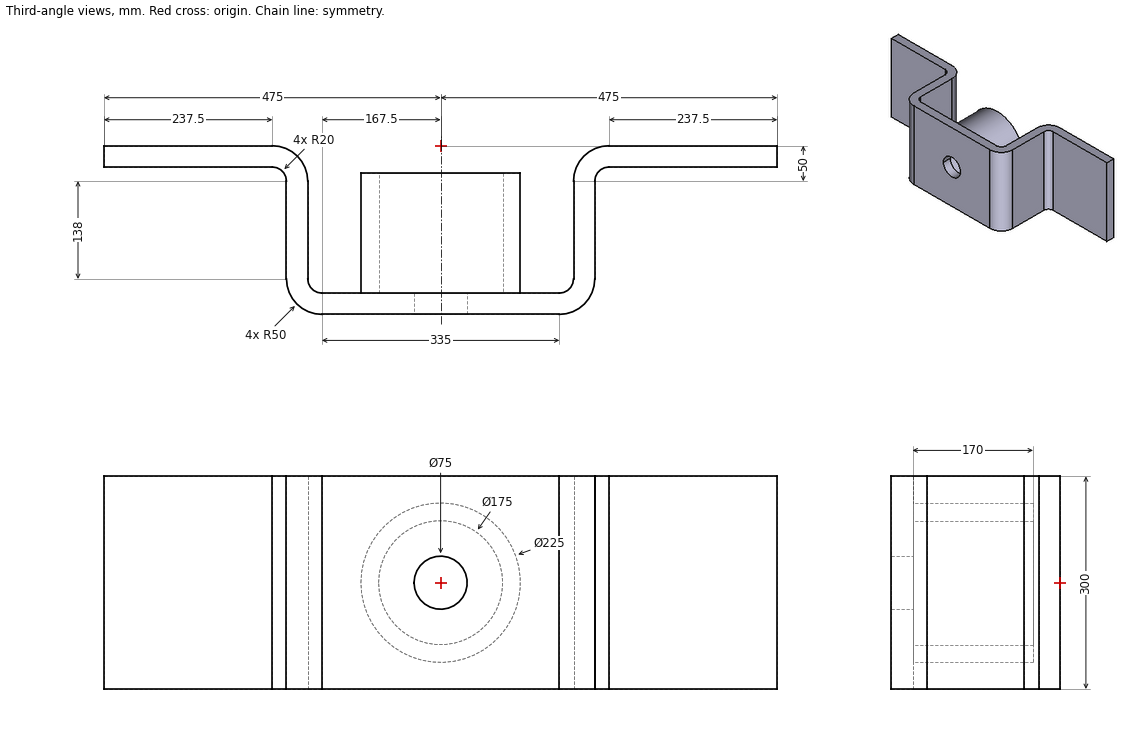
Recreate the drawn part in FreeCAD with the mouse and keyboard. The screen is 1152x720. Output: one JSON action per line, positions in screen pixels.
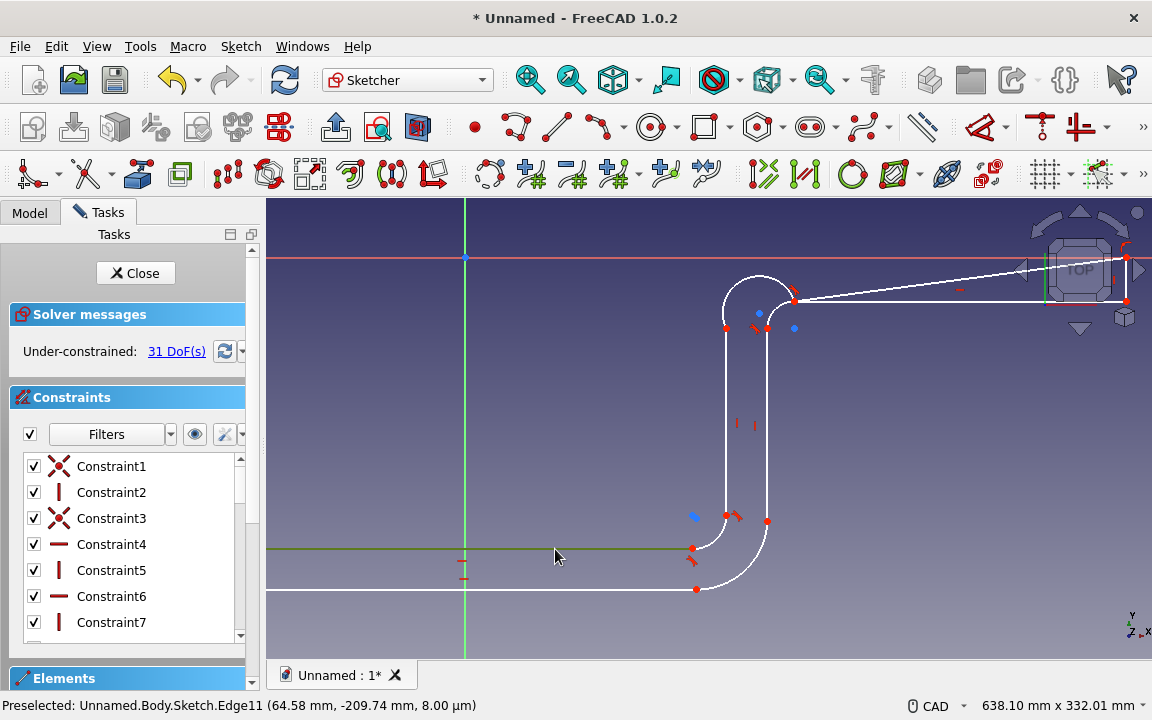
{"action": "scroll", "coordinate": [742, 432], "scroll_direction": "down", "scroll_amount": 5}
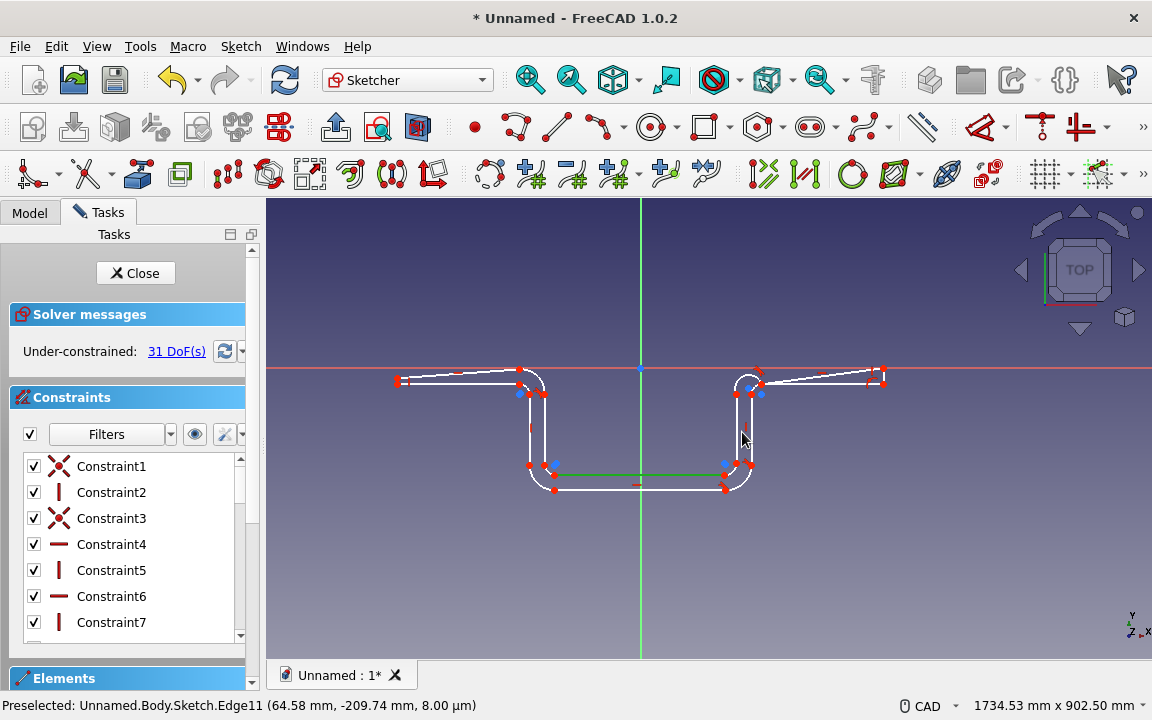
{"action": "scroll", "coordinate": [546, 470], "scroll_direction": "up", "scroll_amount": 6}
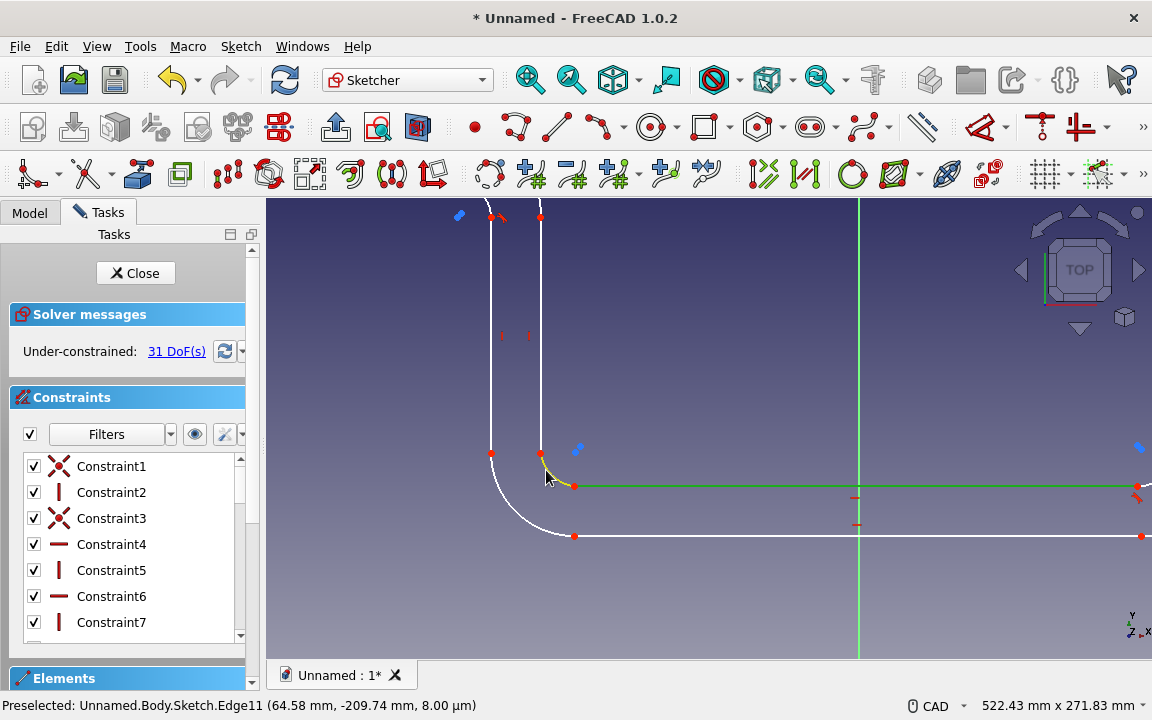
{"action": "left_click", "coordinate": [546, 467]}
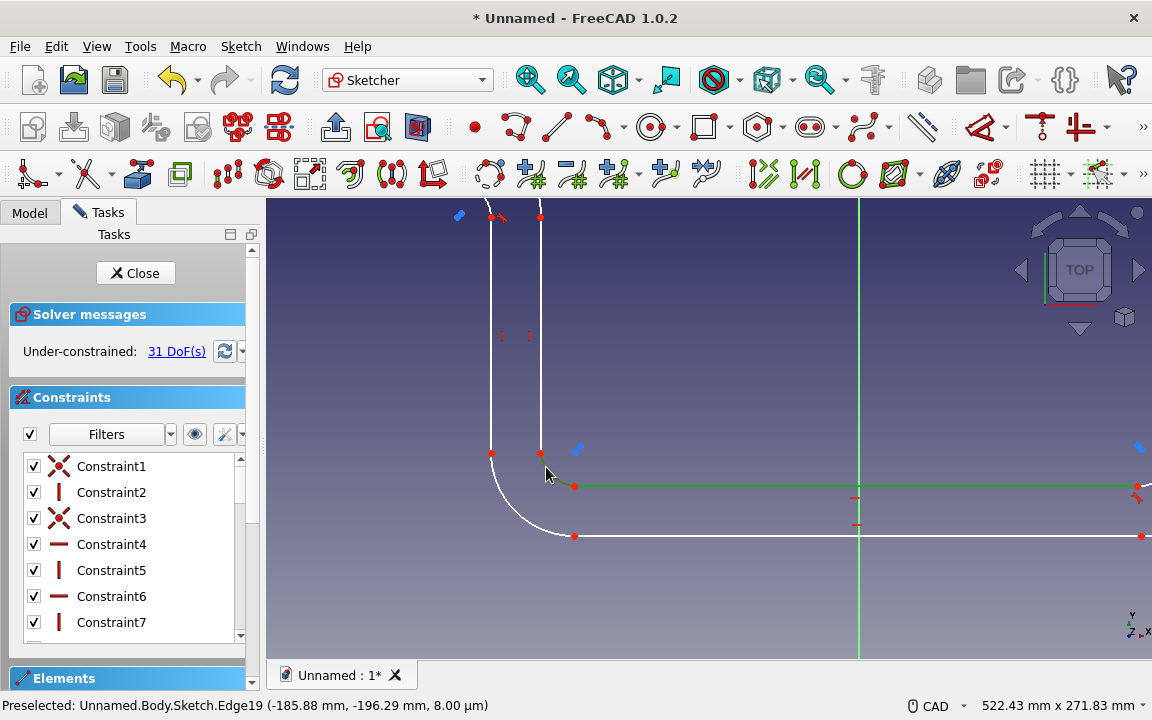
{"action": "key", "text": "t"}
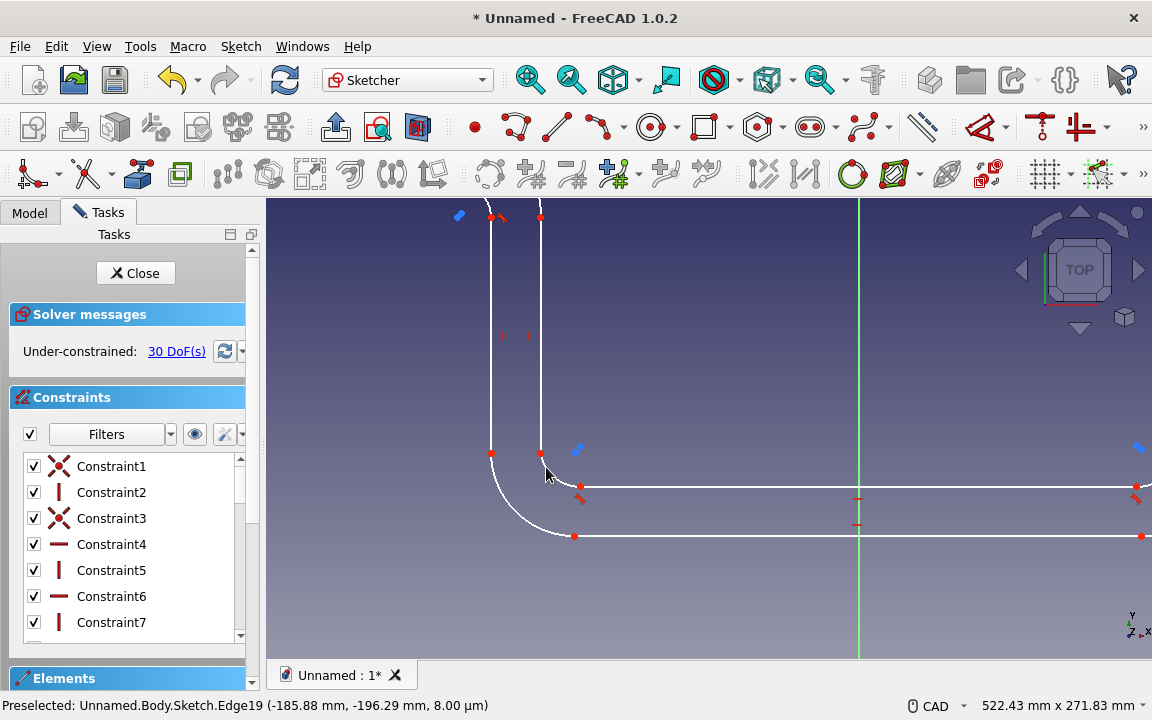
{"action": "left_click", "coordinate": [541, 382]}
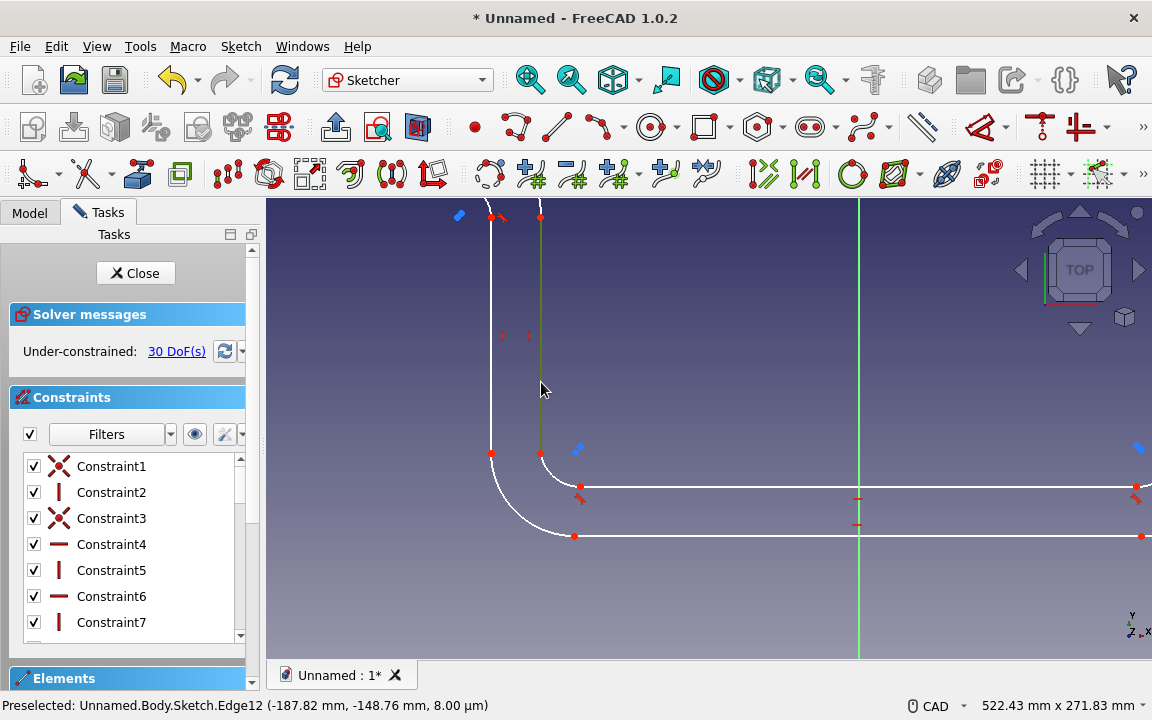
{"action": "left_click", "coordinate": [547, 469]}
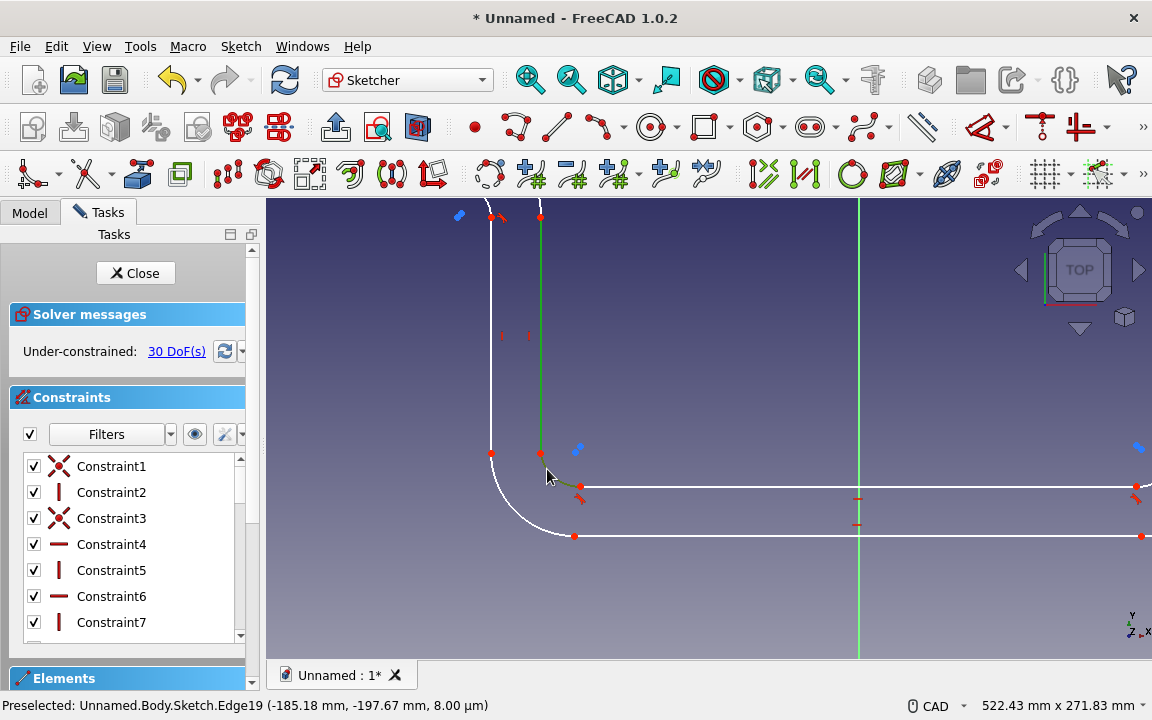
{"action": "key", "text": "t"}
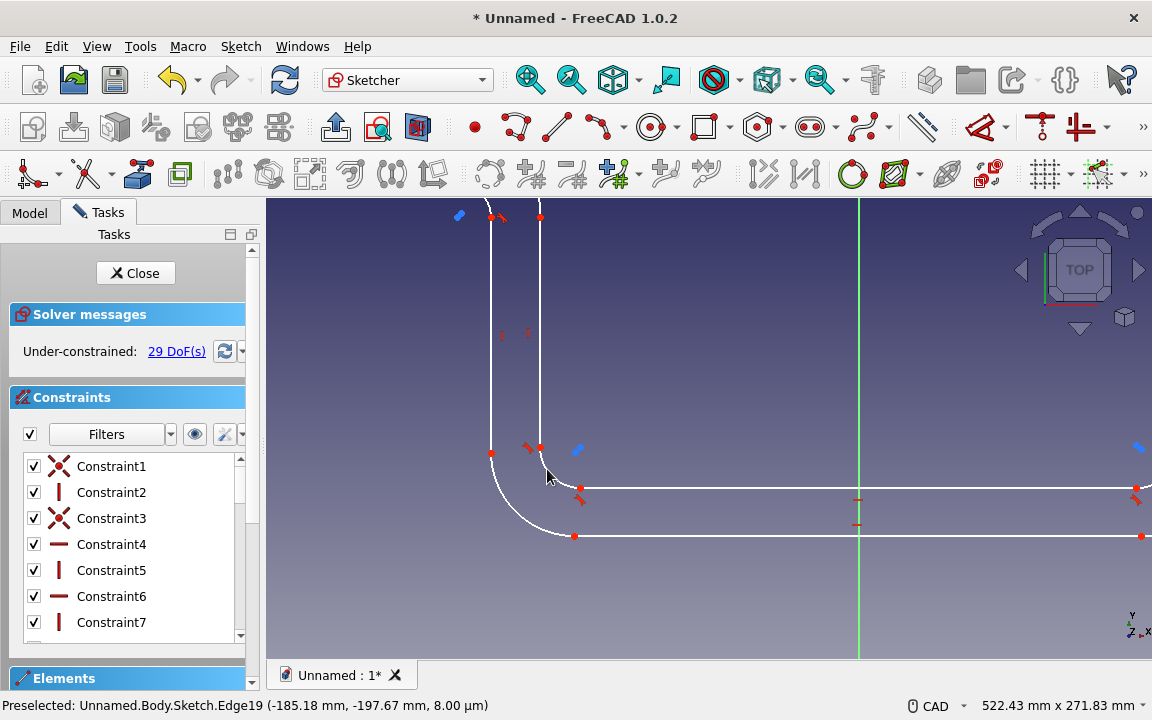
{"action": "scroll", "coordinate": [546, 470], "scroll_direction": "down", "scroll_amount": 6}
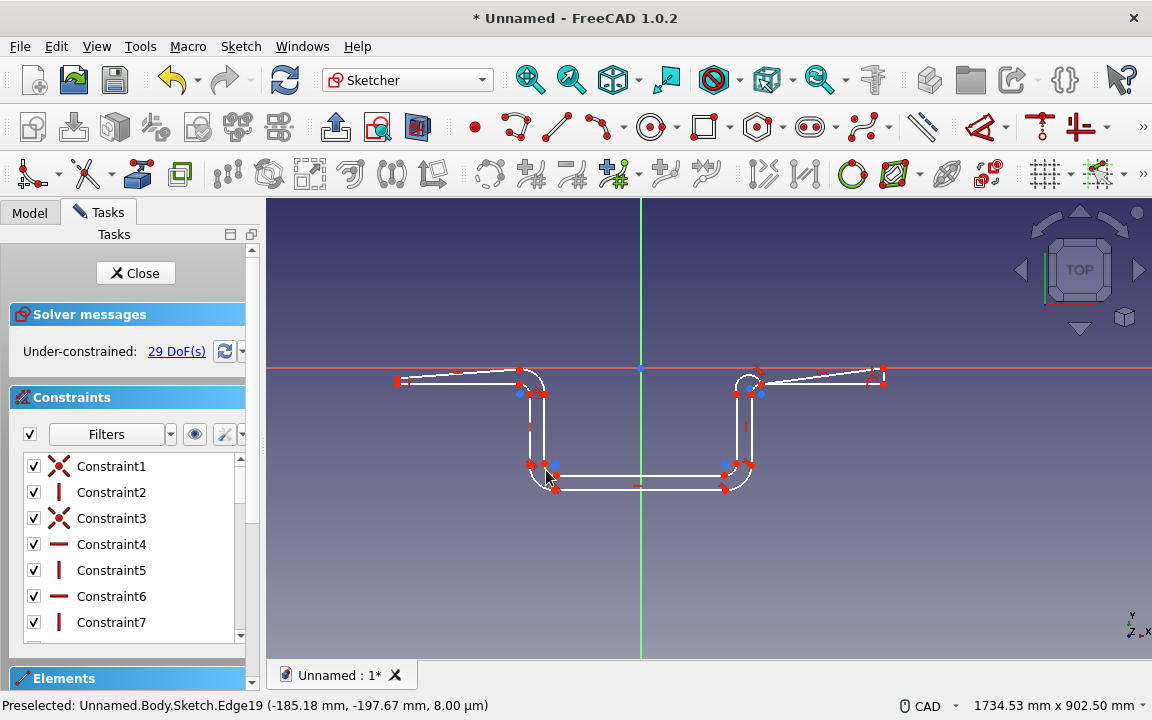
{"action": "scroll", "coordinate": [483, 372], "scroll_direction": "up", "scroll_amount": 7}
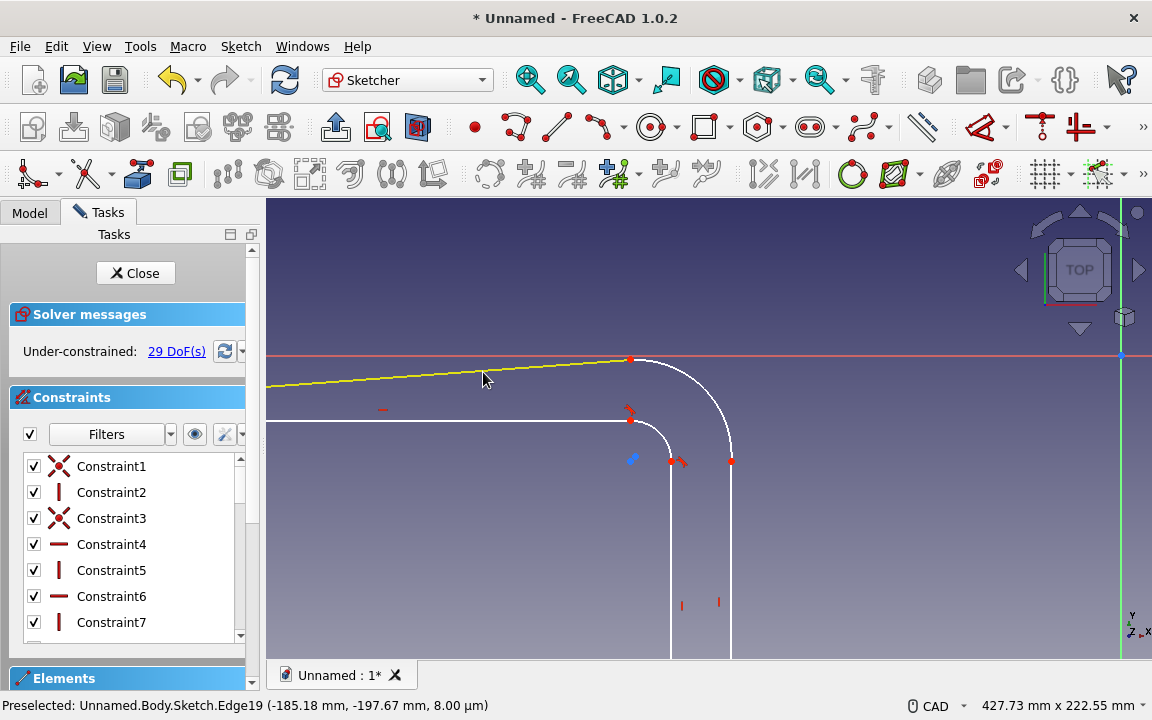
{"action": "left_click", "coordinate": [482, 371]}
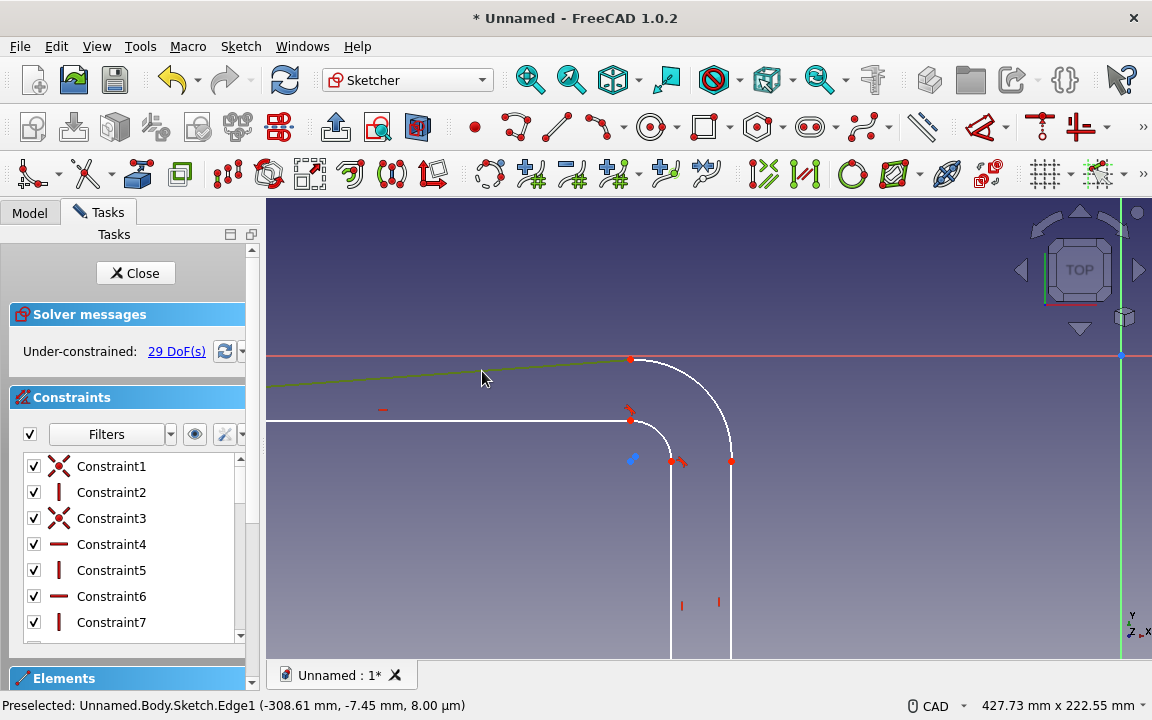
{"action": "key", "text": "h"}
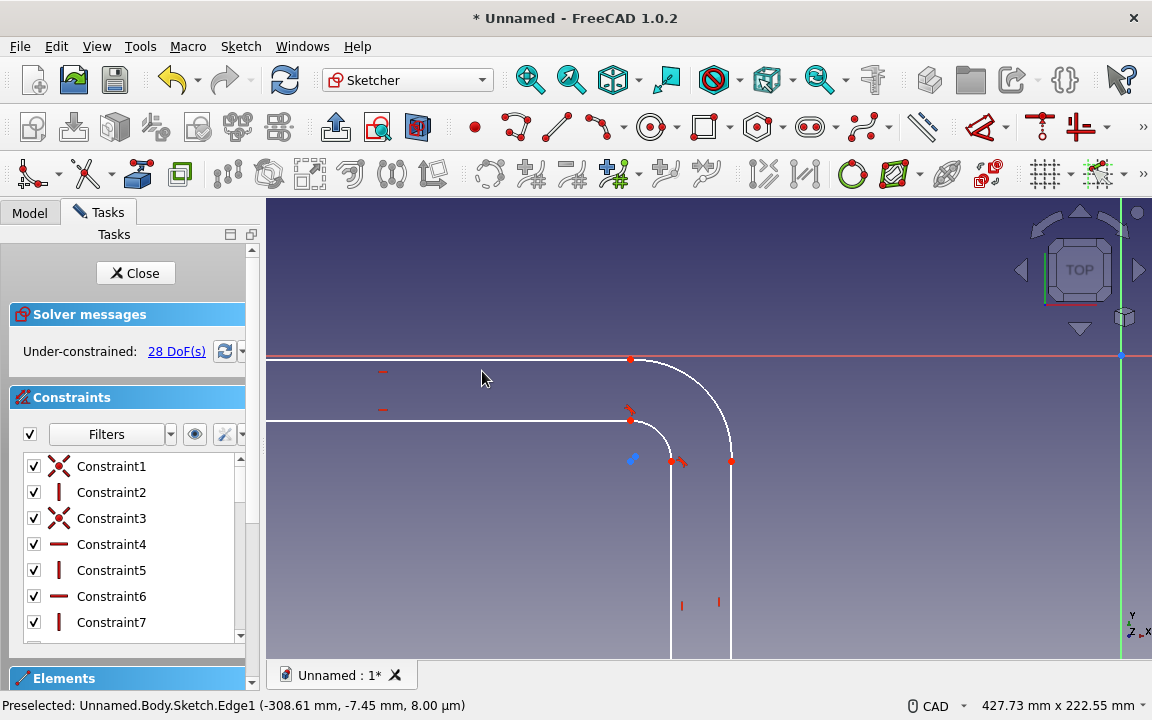
{"action": "scroll", "coordinate": [483, 372], "scroll_direction": "down", "scroll_amount": 7}